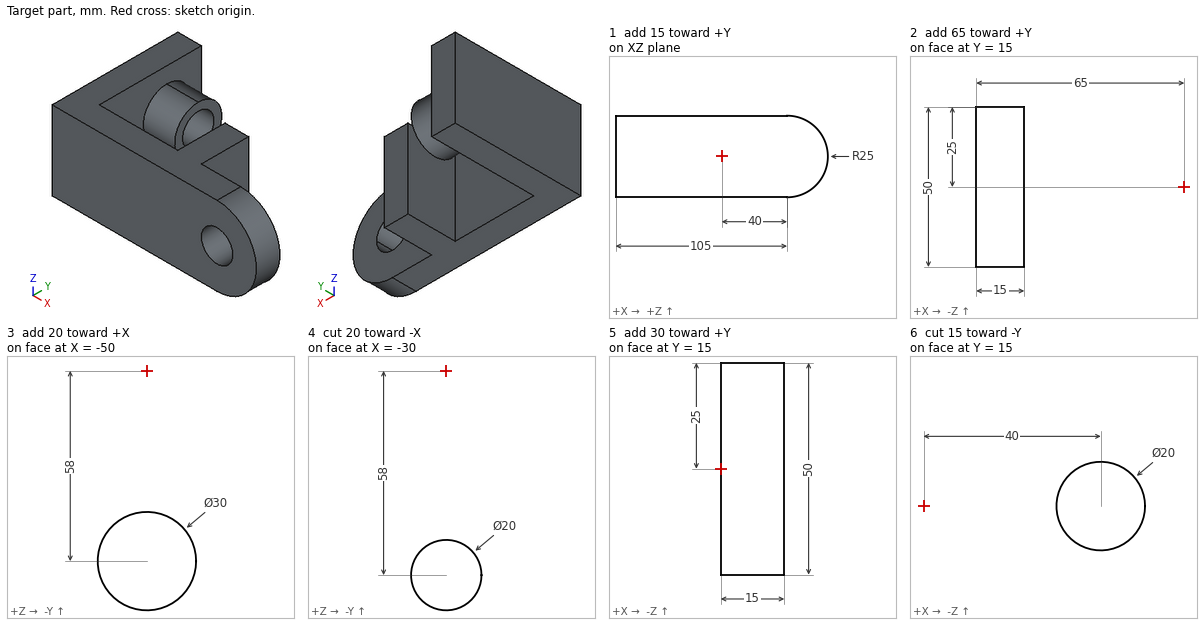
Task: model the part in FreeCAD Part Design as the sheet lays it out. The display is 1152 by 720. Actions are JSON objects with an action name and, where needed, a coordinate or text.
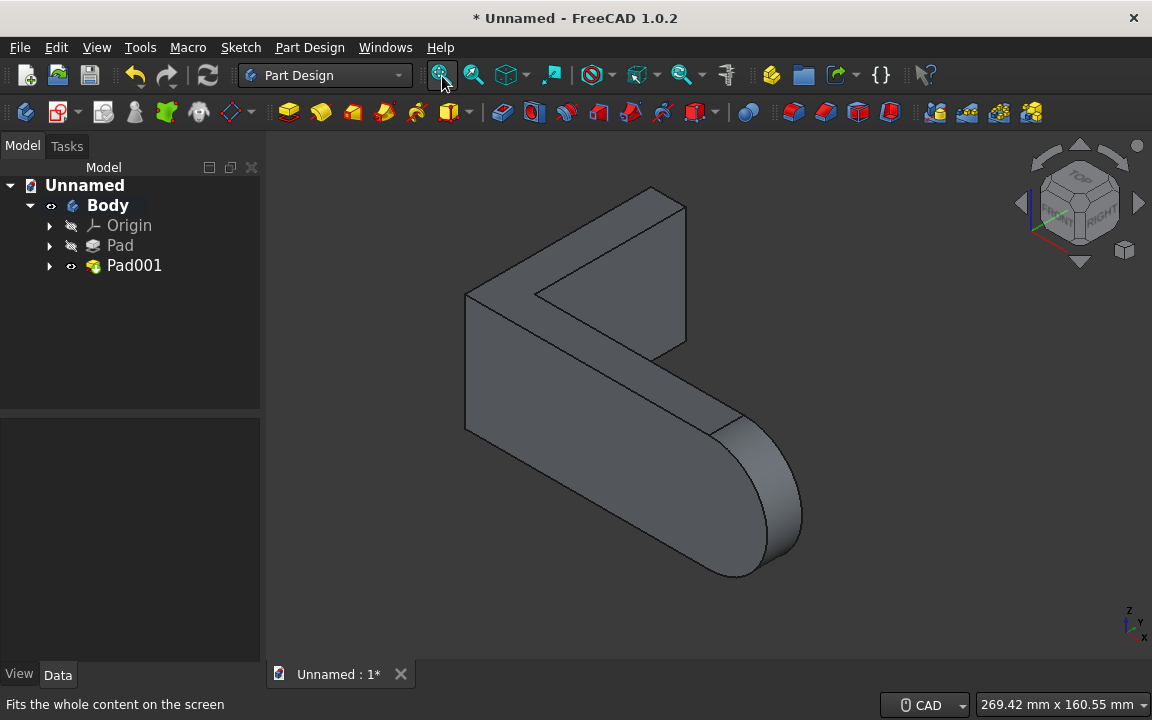
{"action": "left_click", "coordinate": [610, 317]}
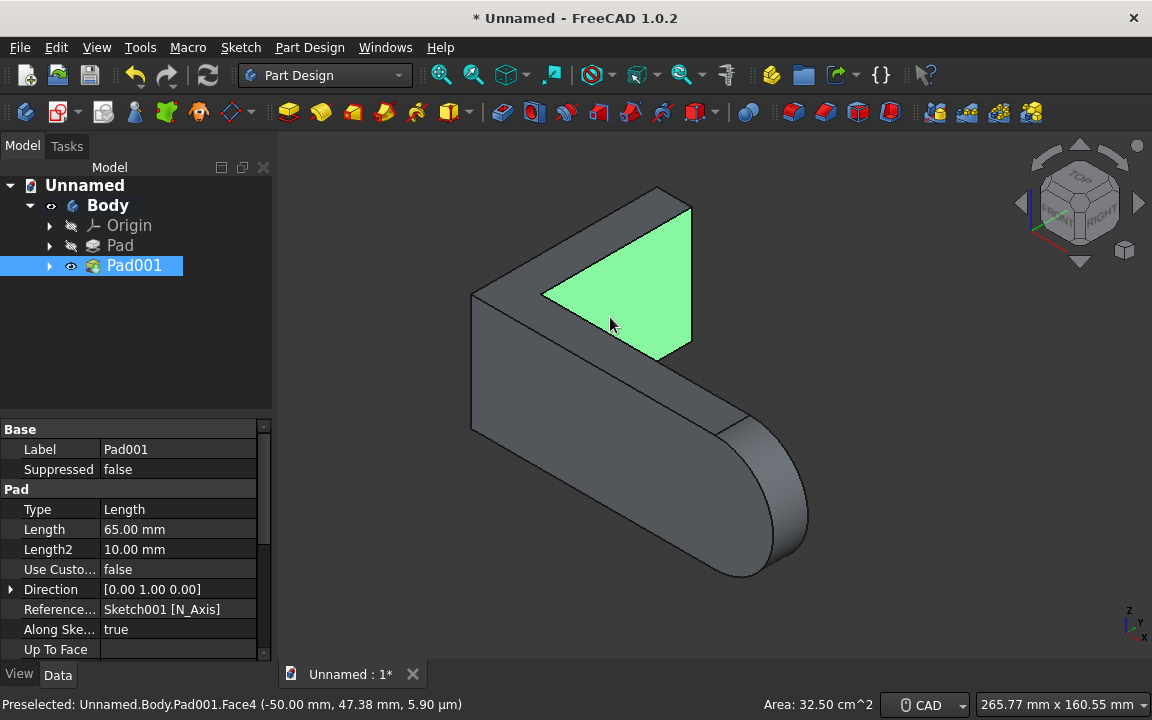
{"action": "left_click", "coordinate": [58, 112]}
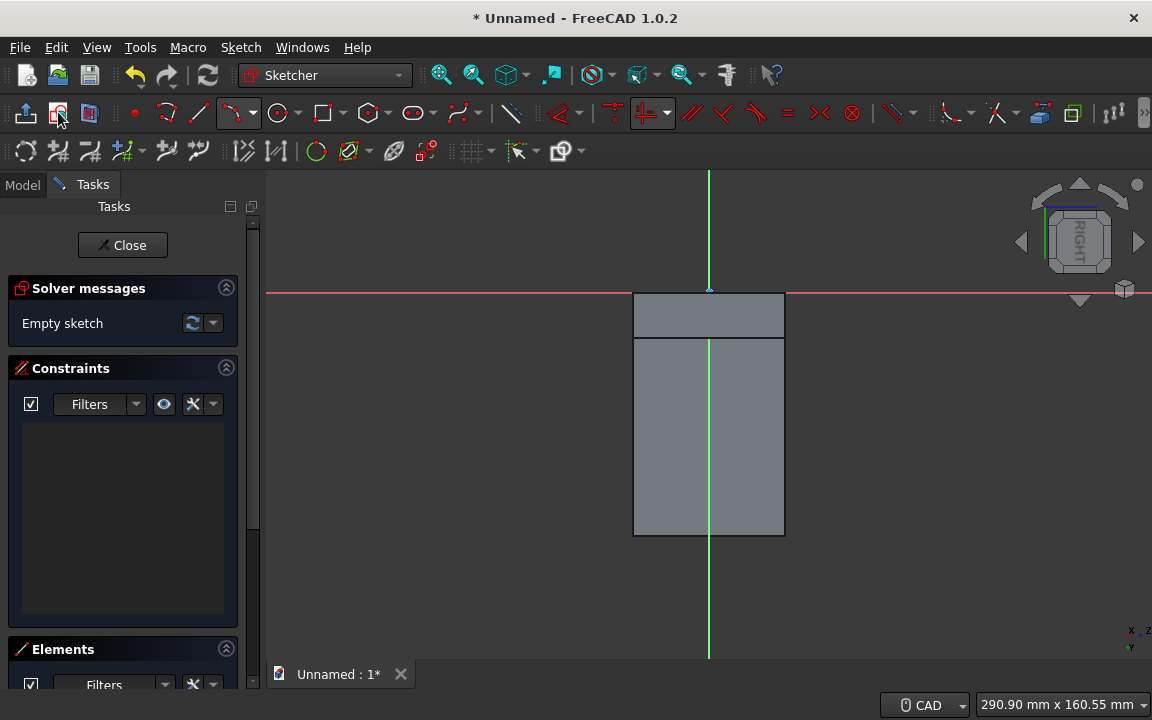
{"action": "scroll", "coordinate": [848, 382], "scroll_direction": "up", "scroll_amount": 2}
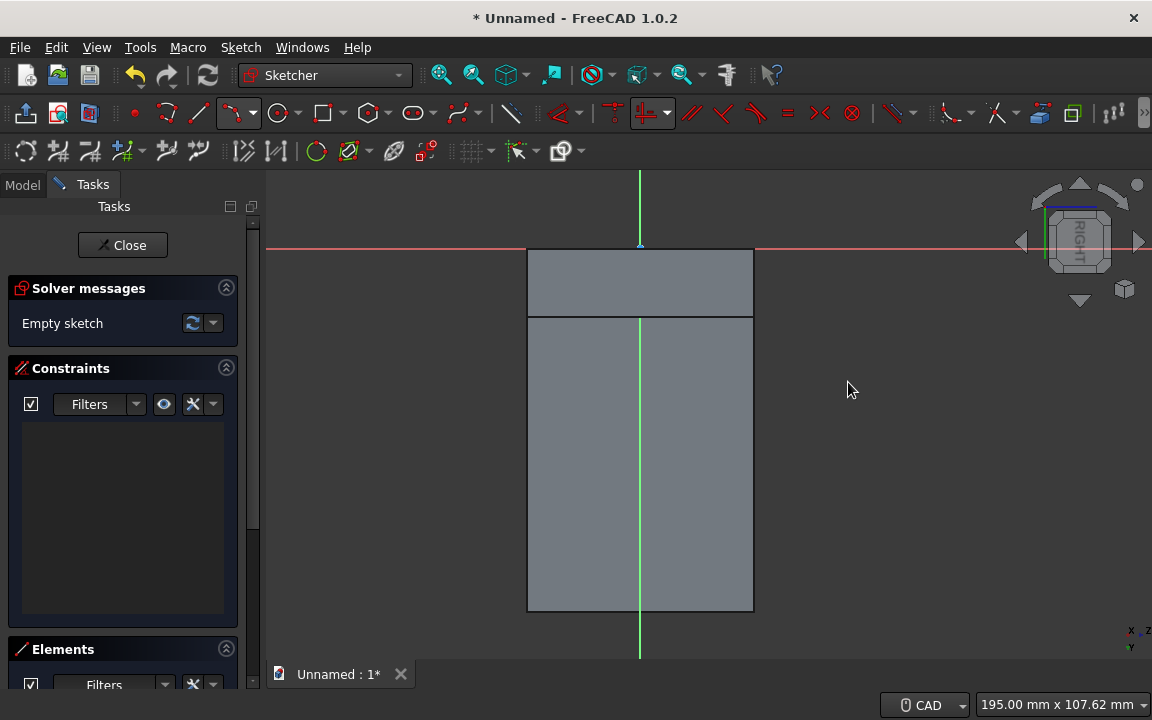
{"action": "left_click", "coordinate": [278, 114]}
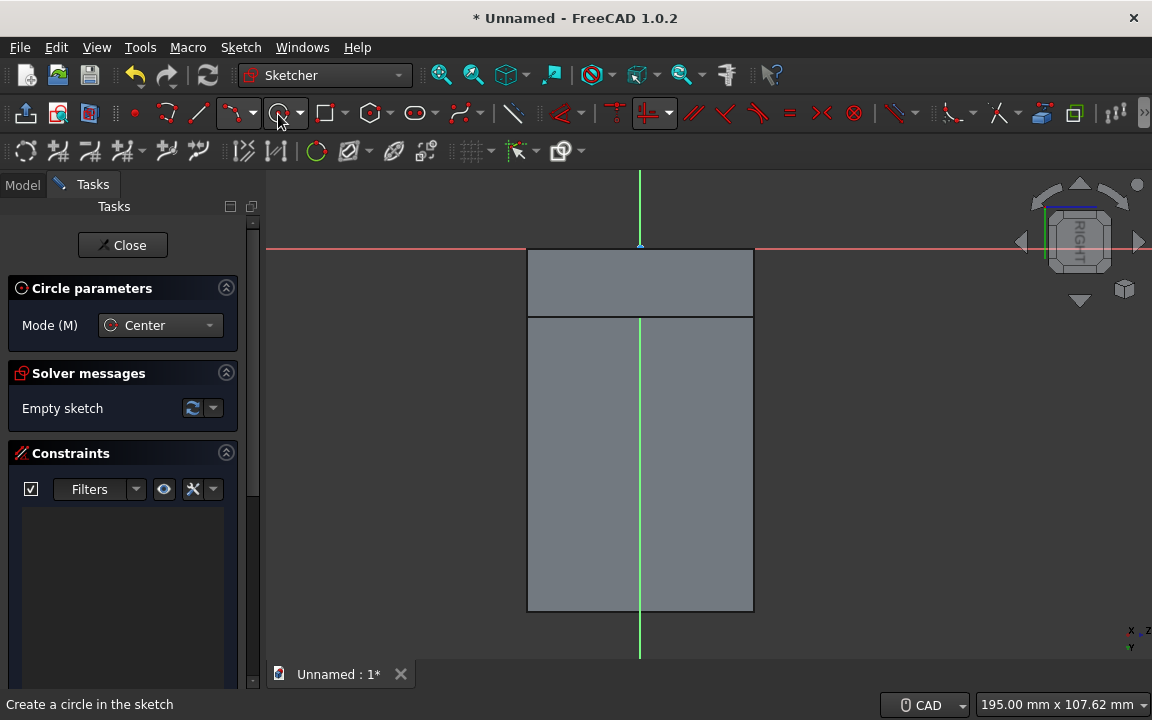
{"action": "left_click", "coordinate": [640, 512]}
{"action": "mouse_move", "coordinate": [689, 464]}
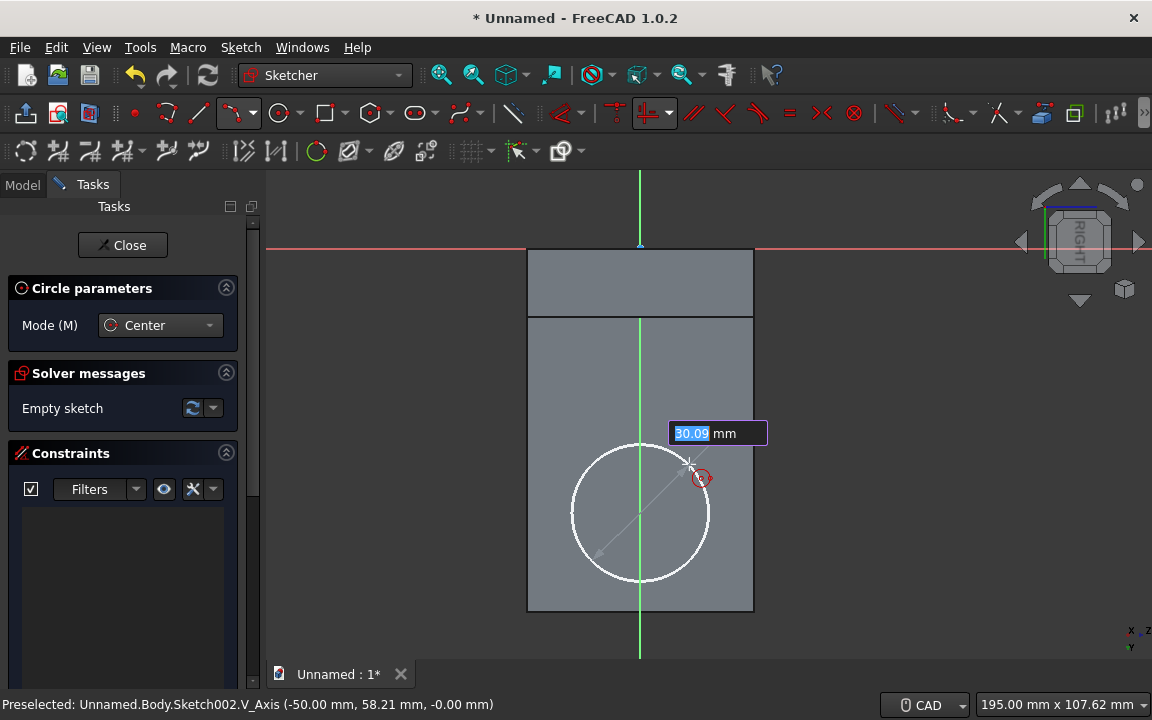
{"action": "type", "text": "30"}
{"action": "key", "text": "Return"}
{"action": "key", "text": "Escape"}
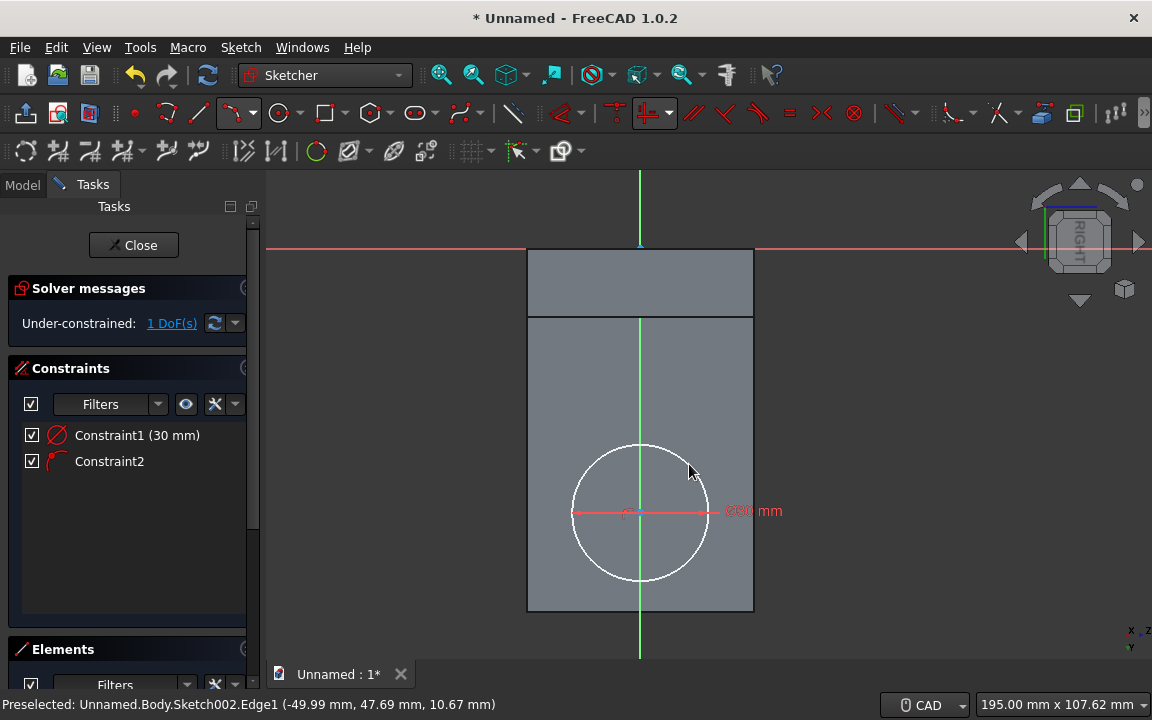
{"action": "left_click", "coordinate": [560, 114]}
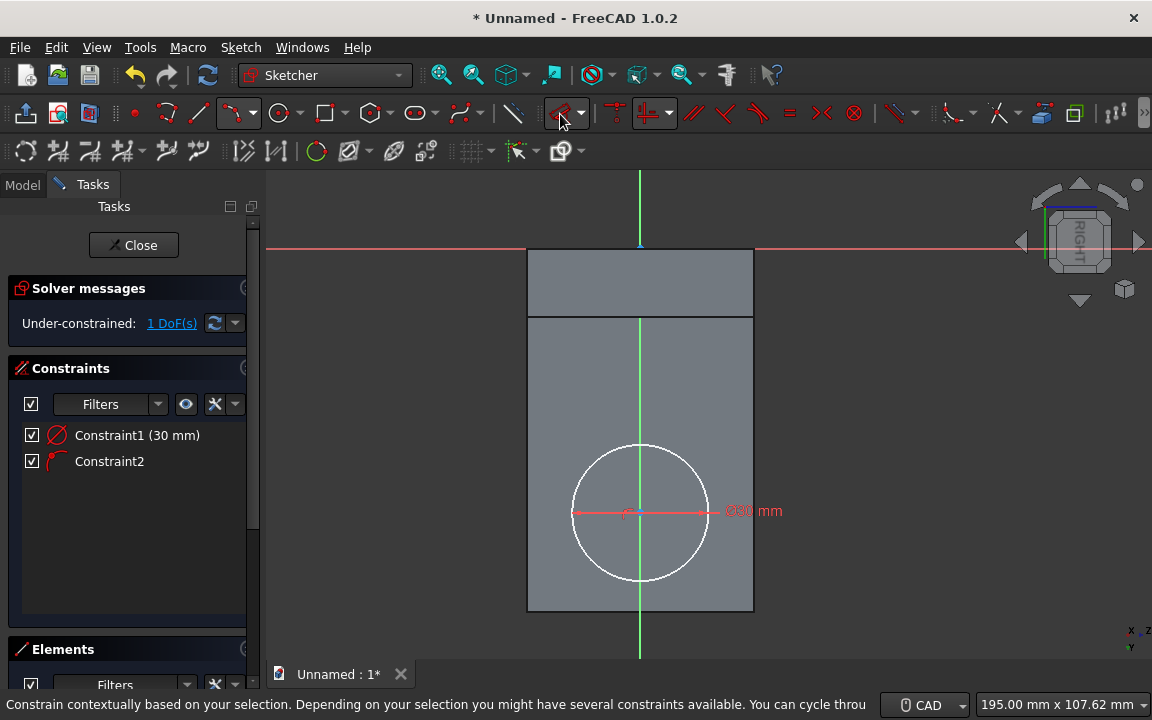
{"action": "left_click", "coordinate": [640, 513]}
{"action": "left_click", "coordinate": [674, 381]}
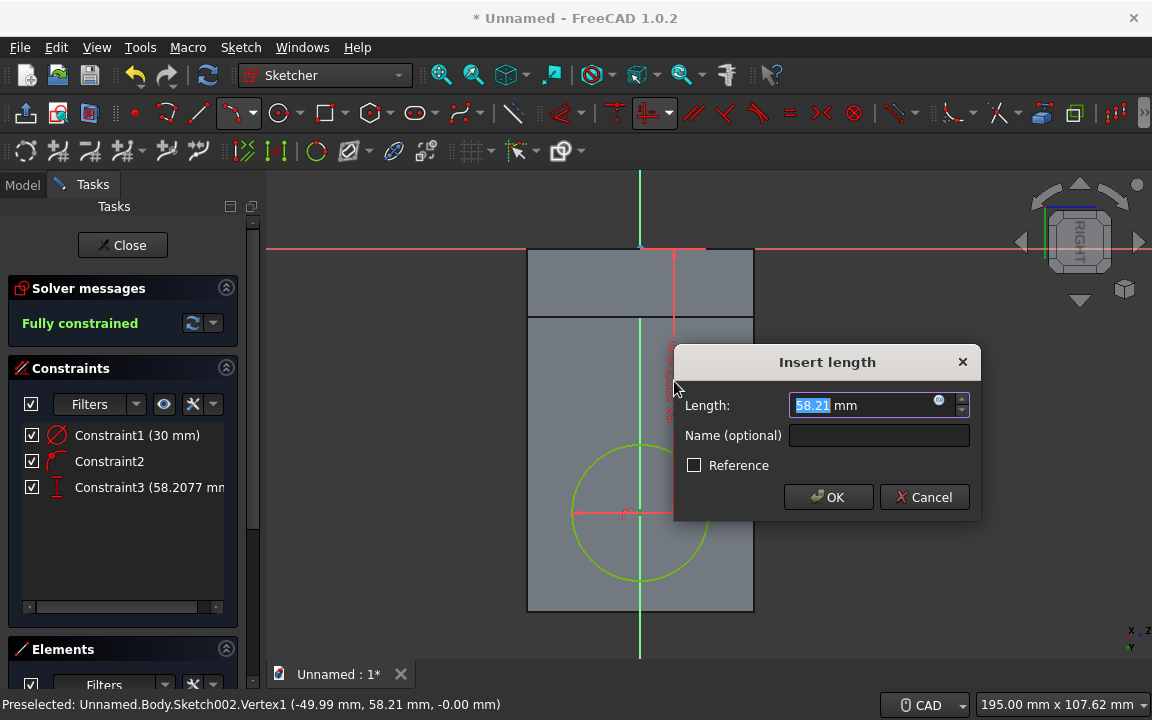
{"action": "type", "text": "58"}
{"action": "key", "text": "Return"}
{"action": "key", "text": "Escape"}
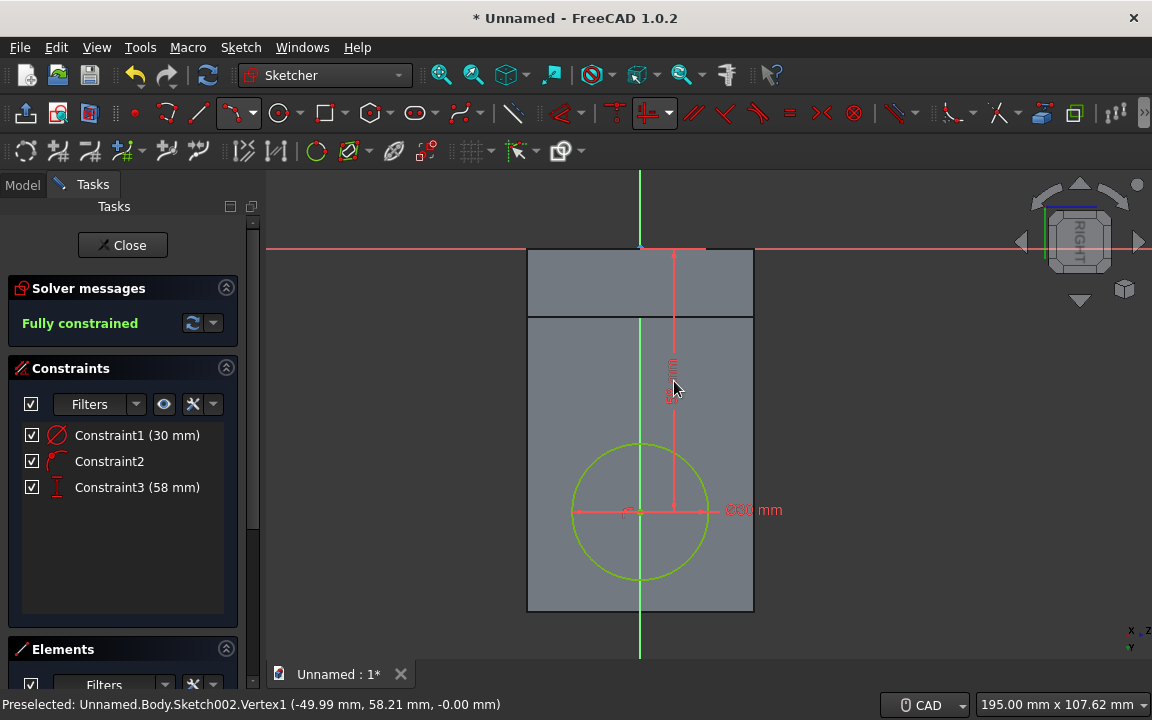
{"action": "left_click", "coordinate": [123, 245]}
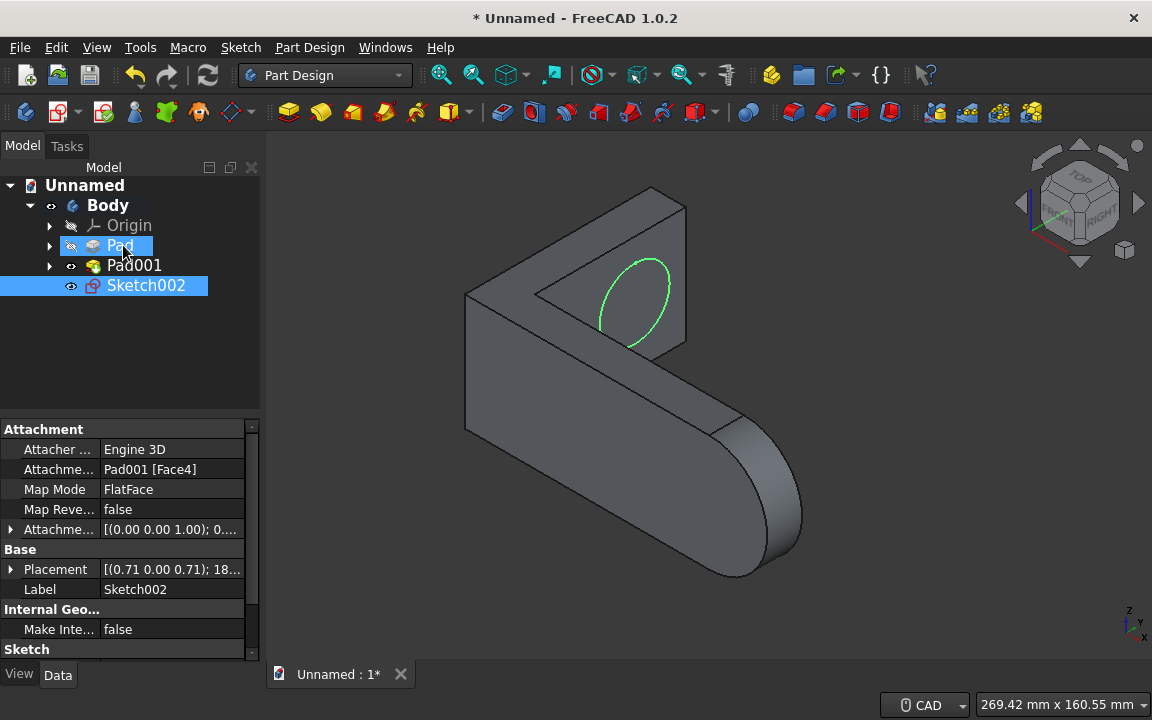
{"action": "left_click", "coordinate": [290, 112]}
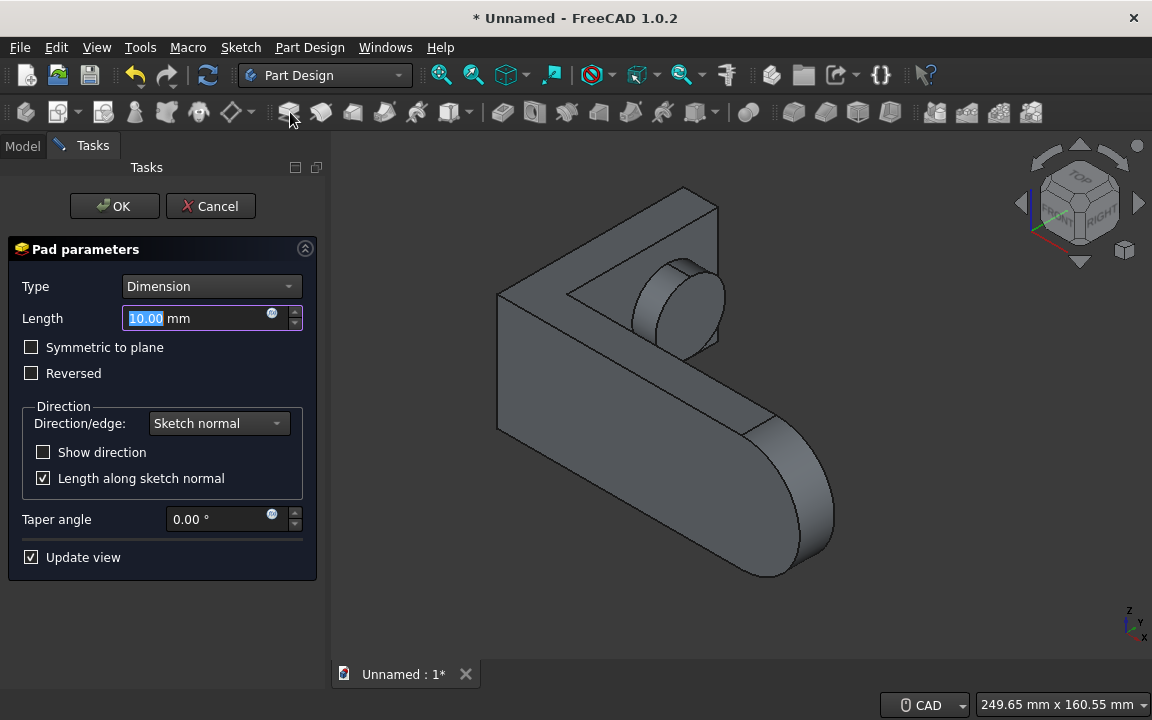
{"action": "type", "text": "20"}
{"action": "key", "text": "Tab"}